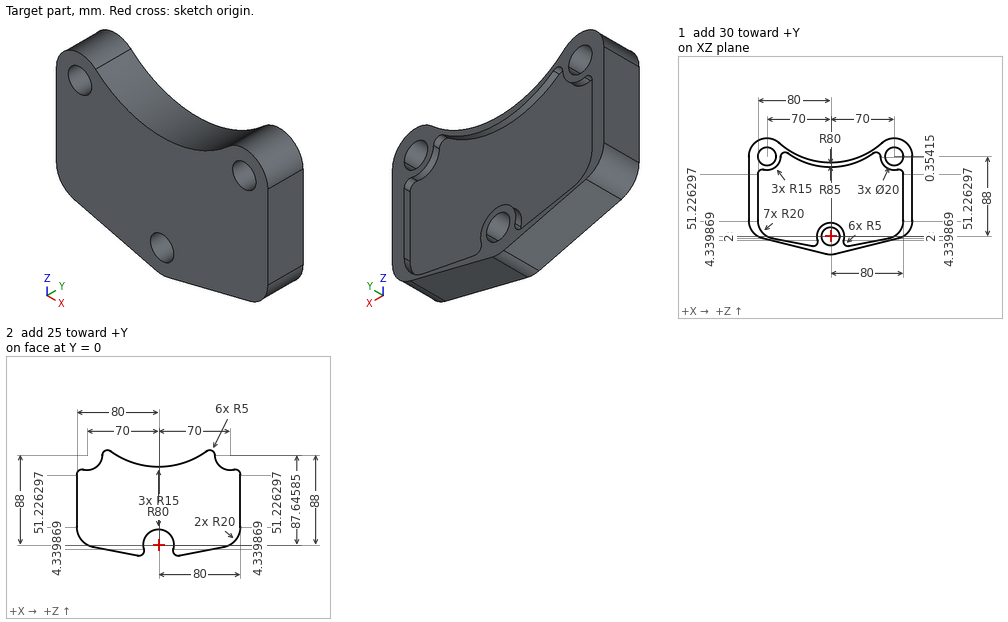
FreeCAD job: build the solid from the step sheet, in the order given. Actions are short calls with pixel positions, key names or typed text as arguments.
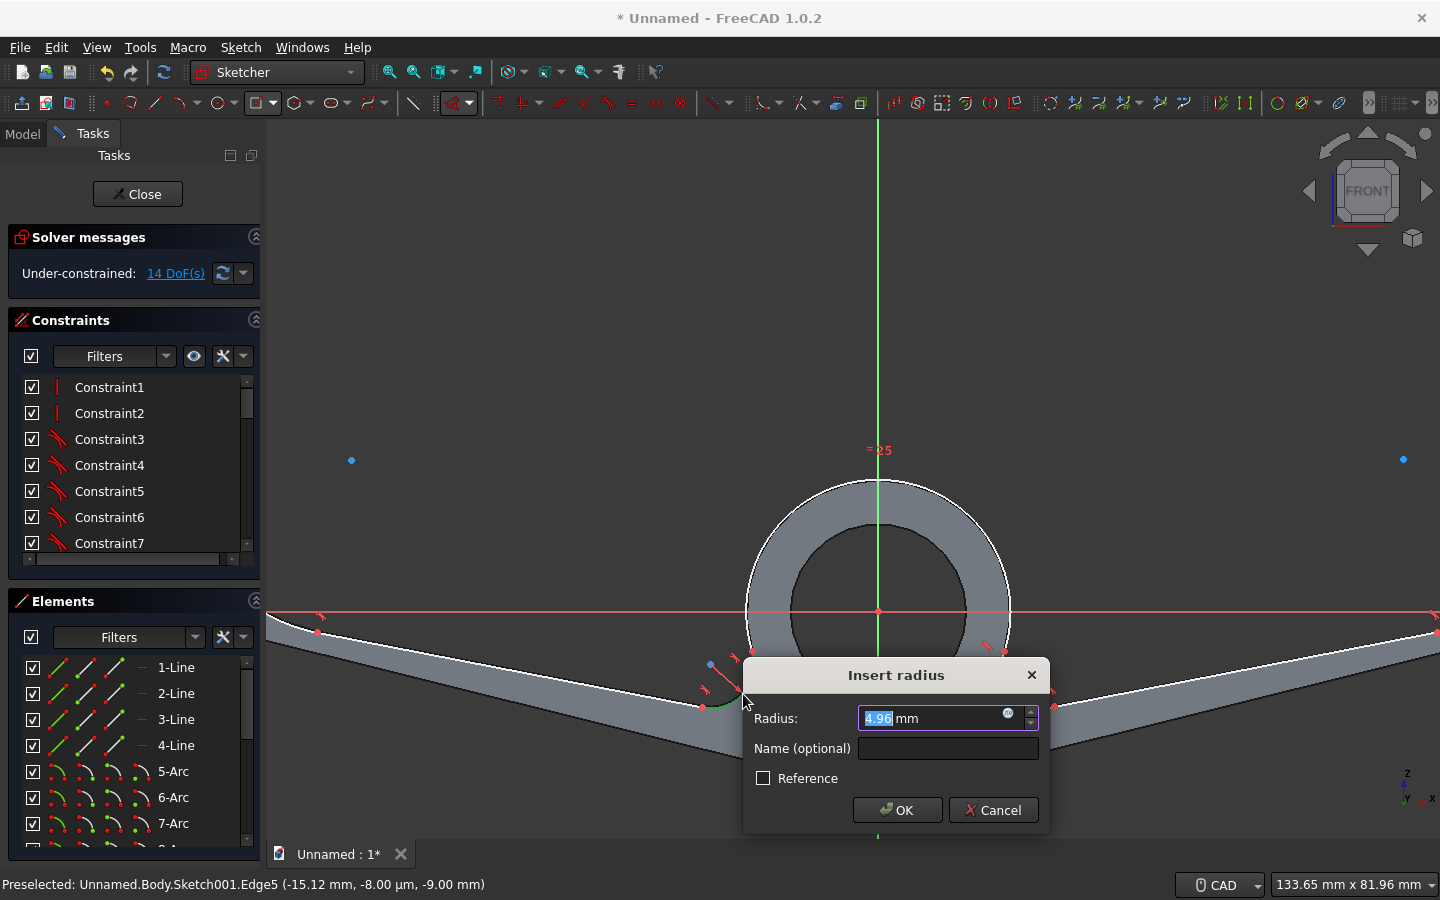
text(5)
key(Return)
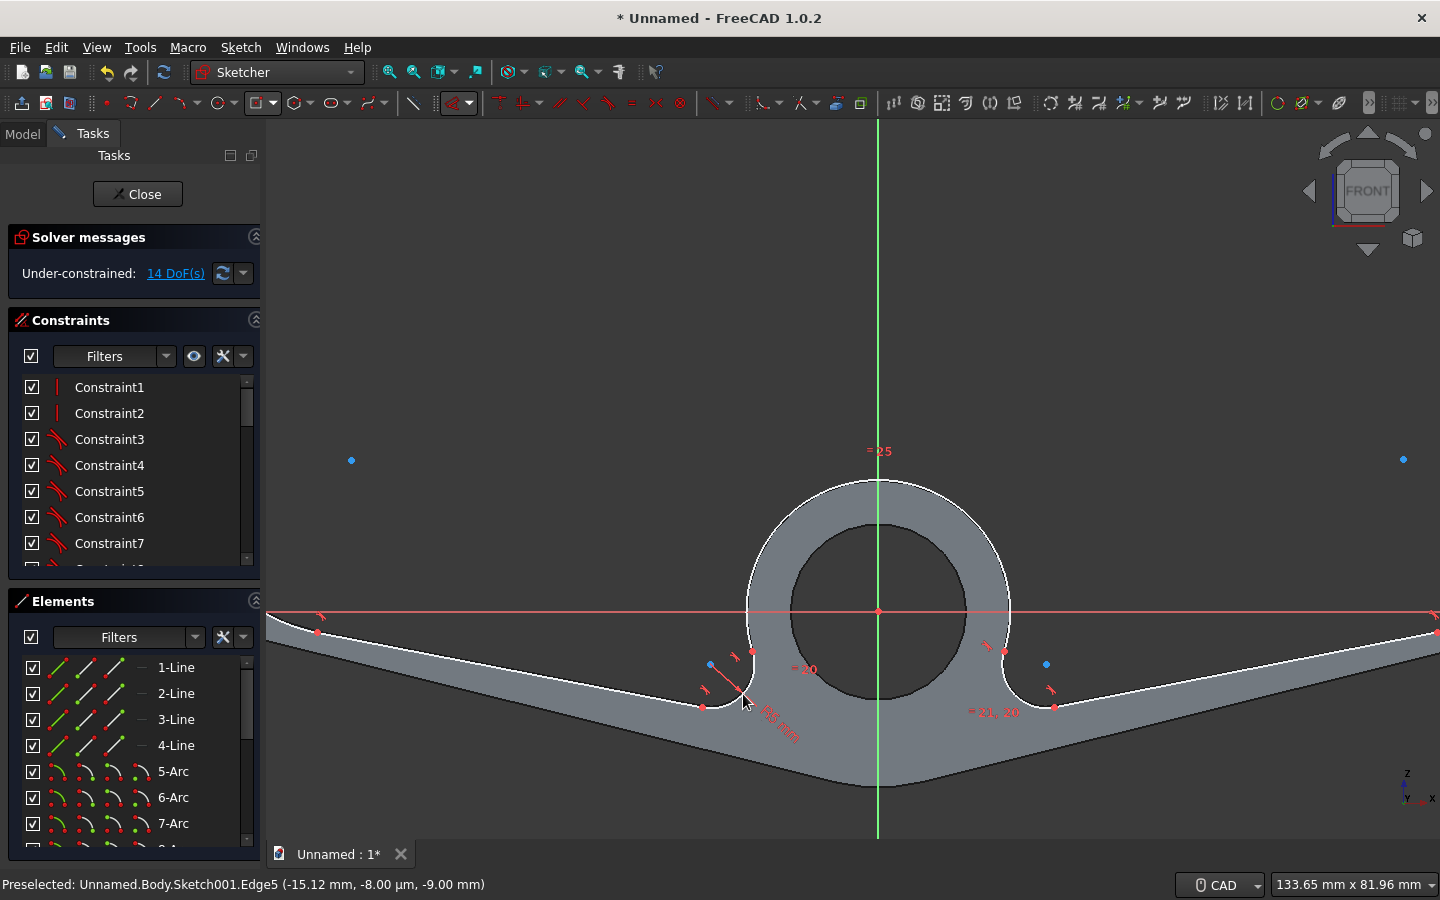
click(968, 515)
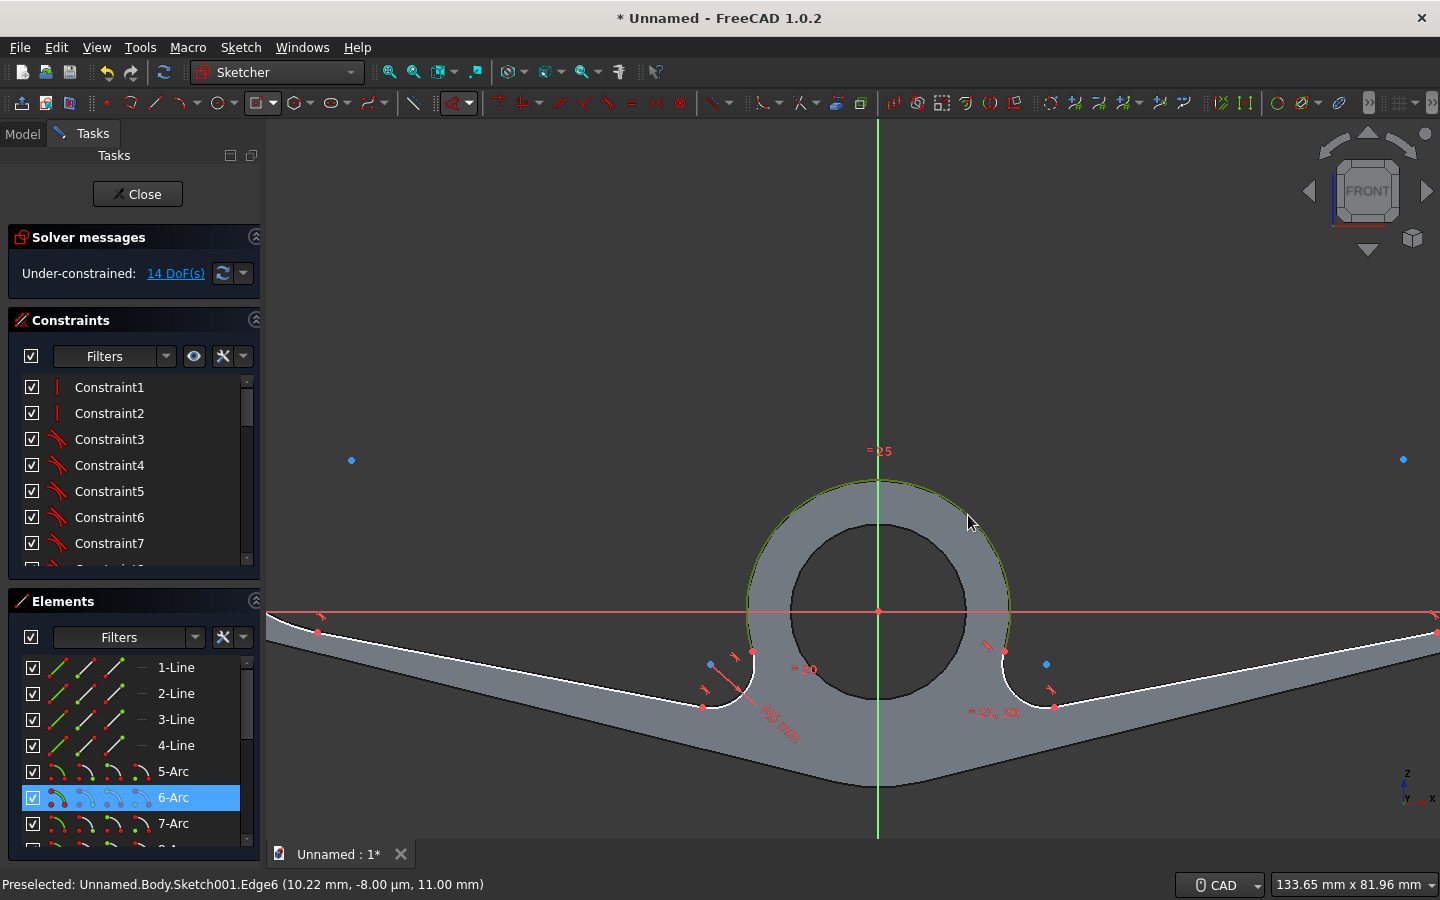
click(472, 104)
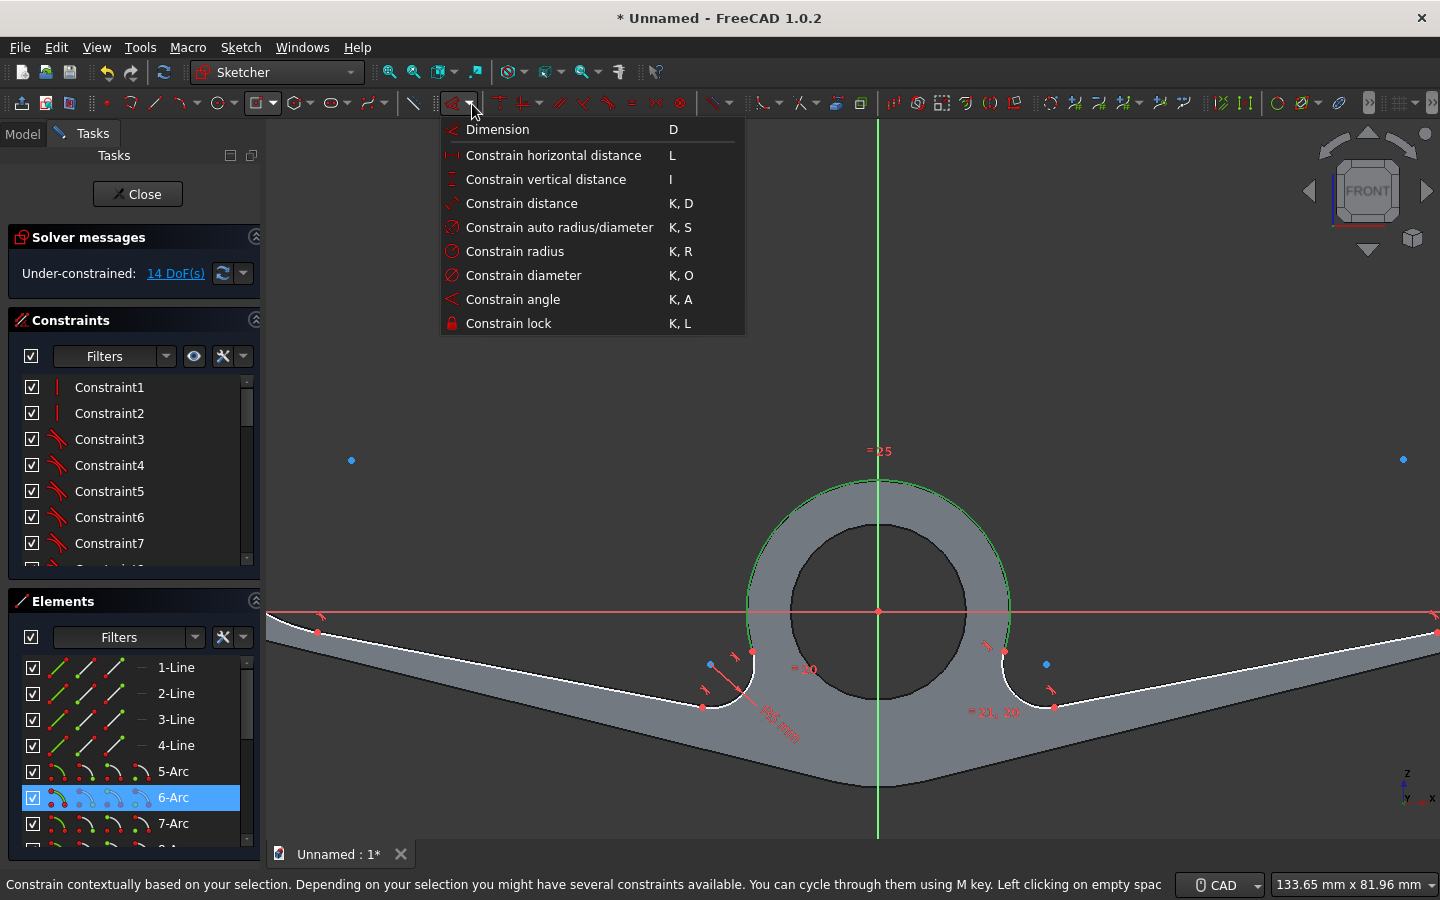
click(593, 251)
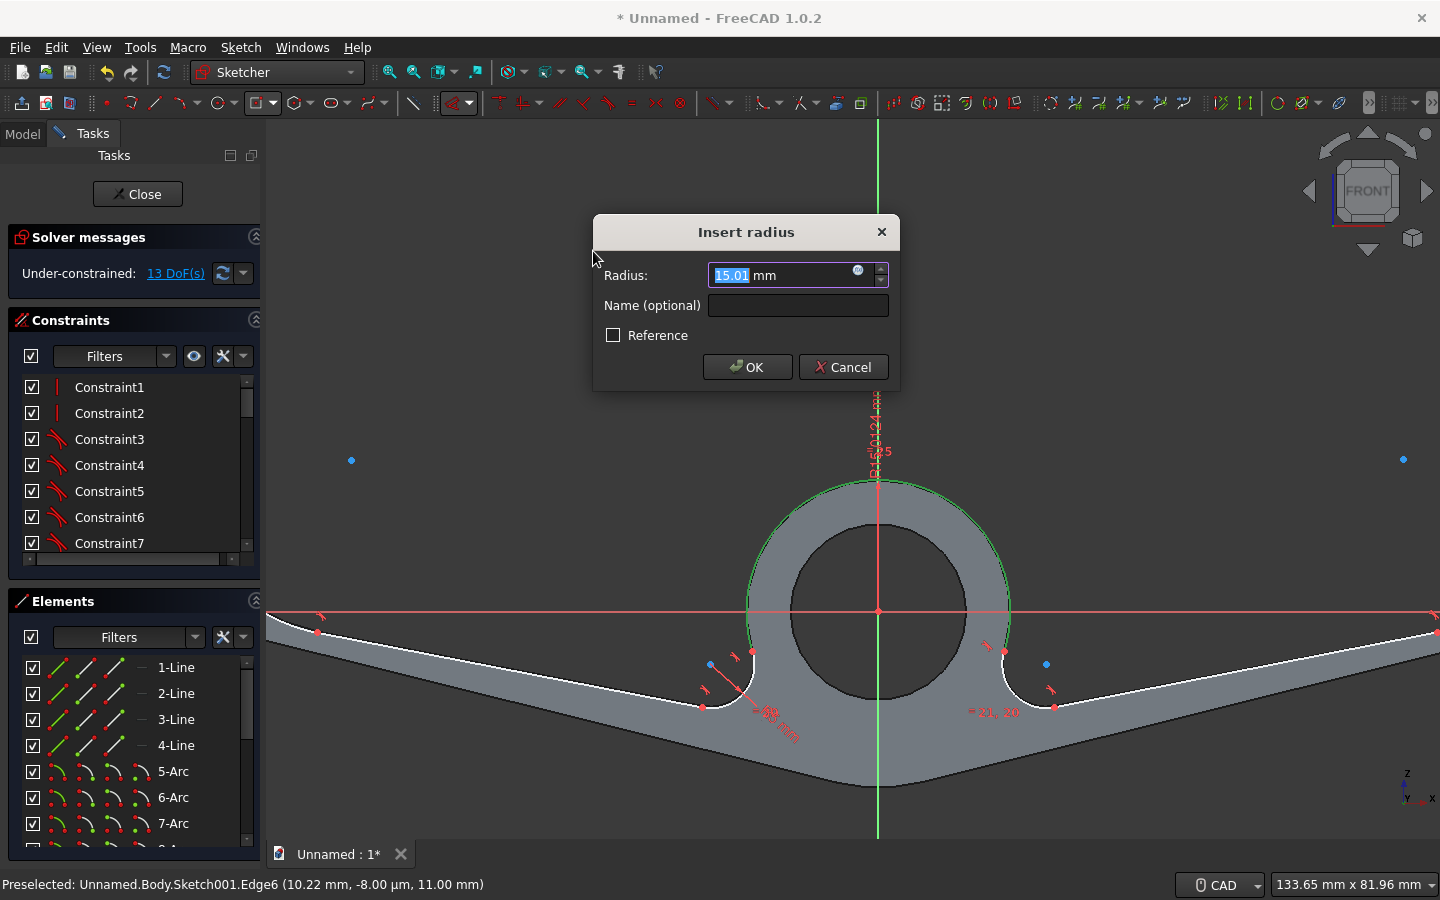
text(15)
key(Return)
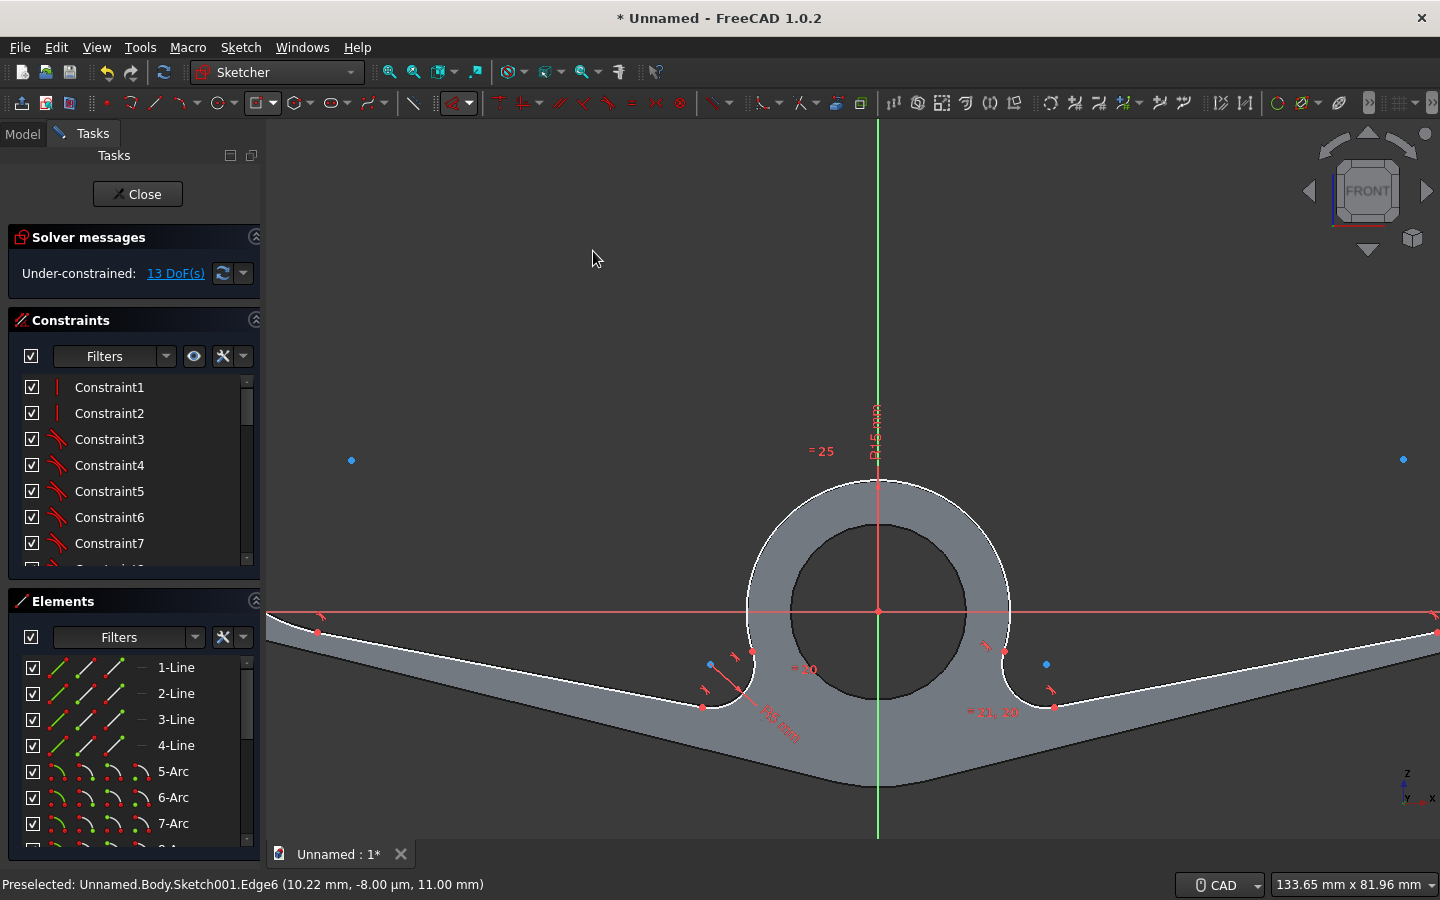
scroll(708, 662, down, 4)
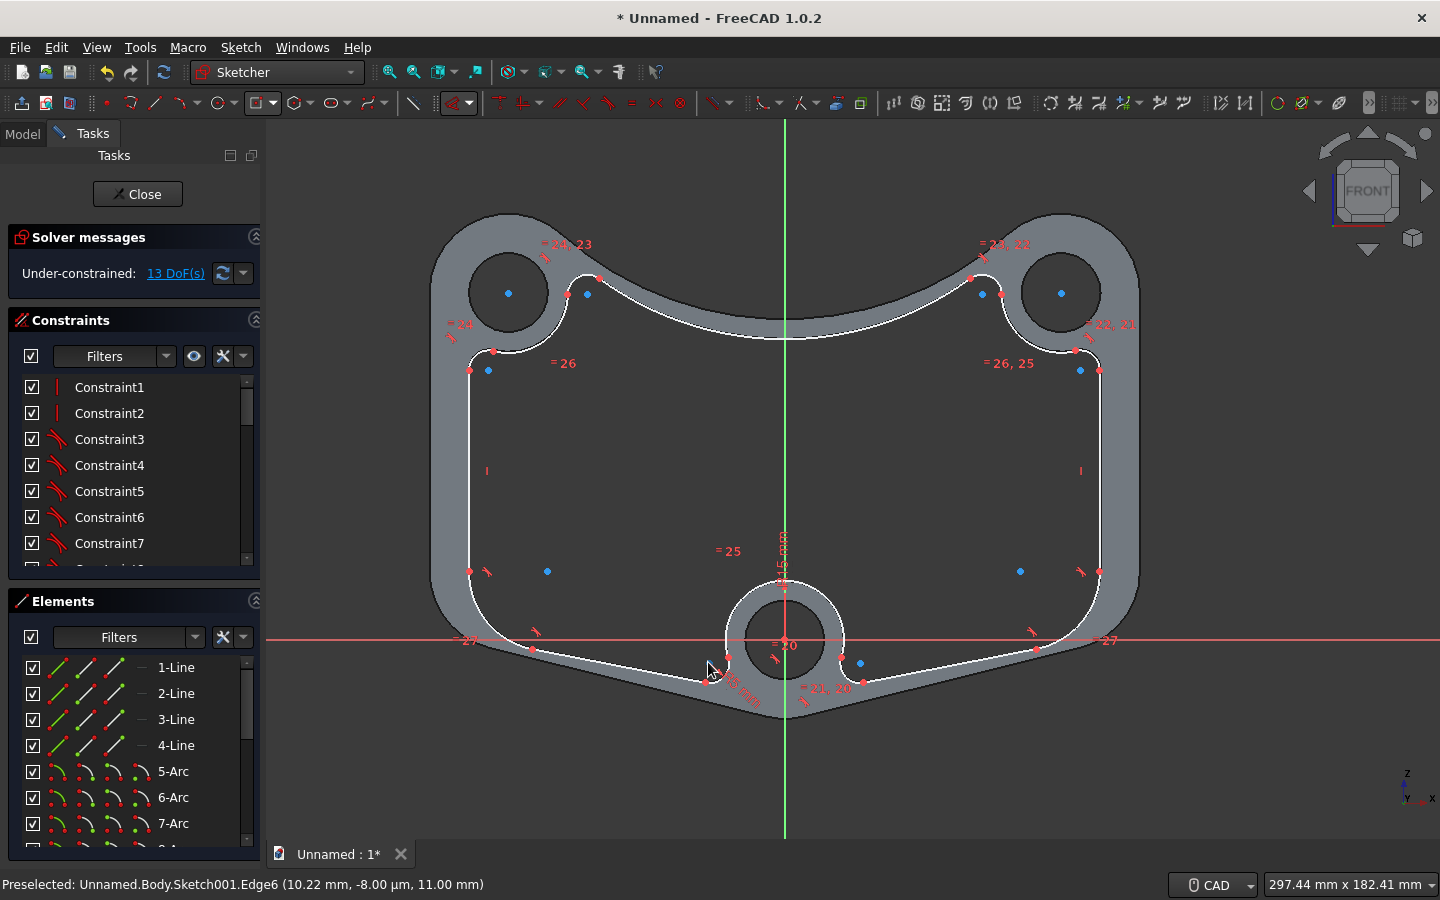
click(1093, 603)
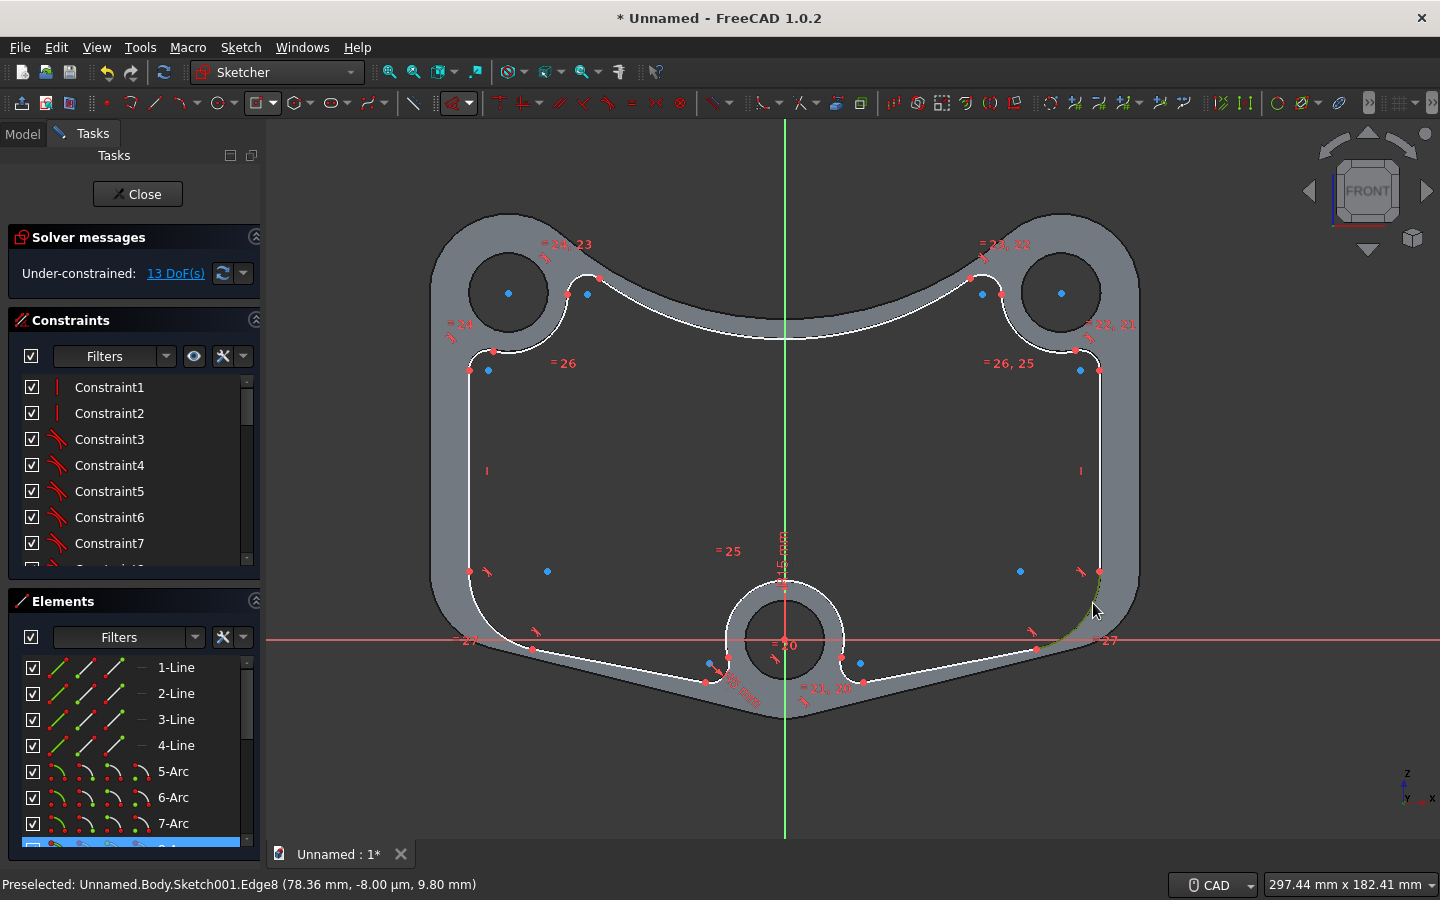
key(k)
key(r)